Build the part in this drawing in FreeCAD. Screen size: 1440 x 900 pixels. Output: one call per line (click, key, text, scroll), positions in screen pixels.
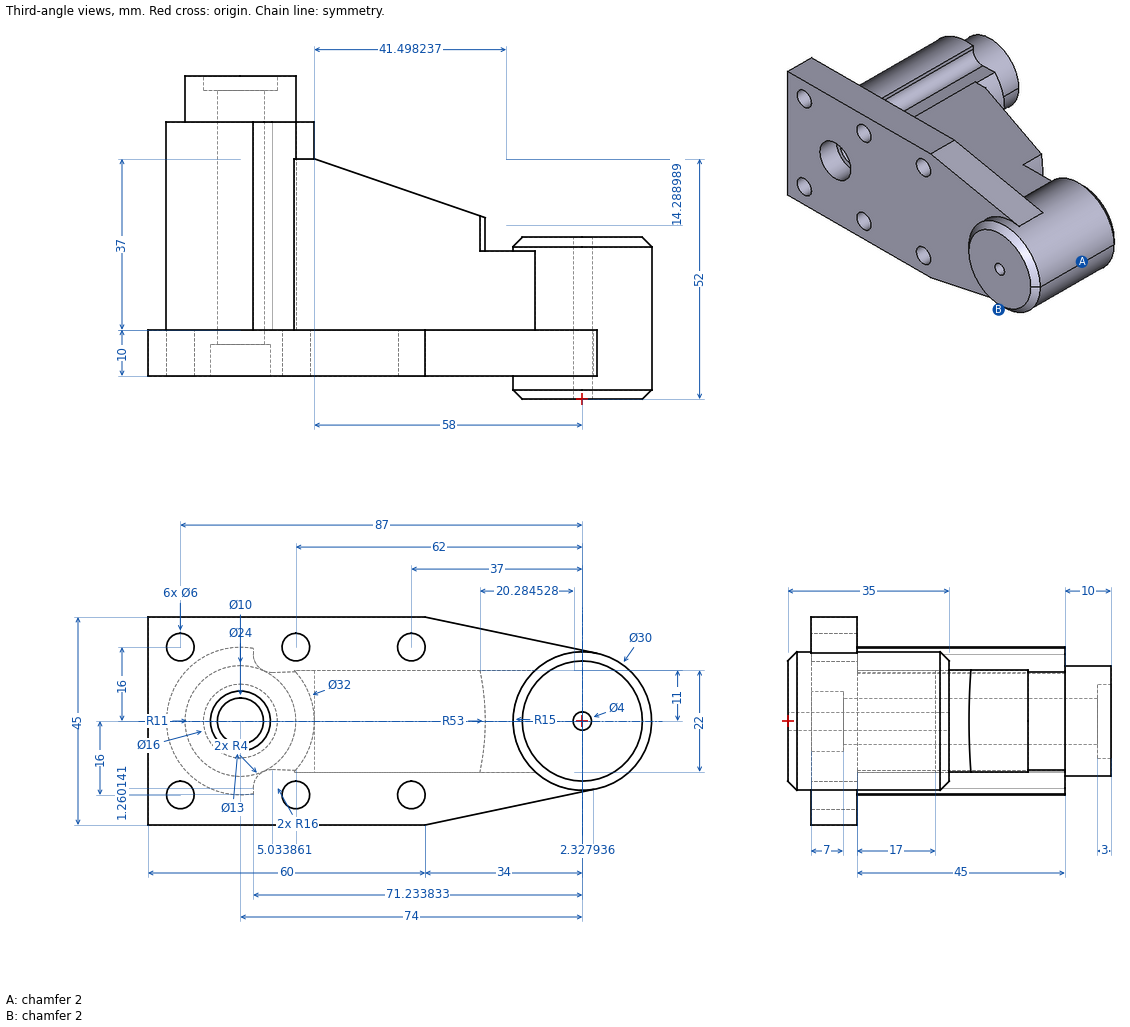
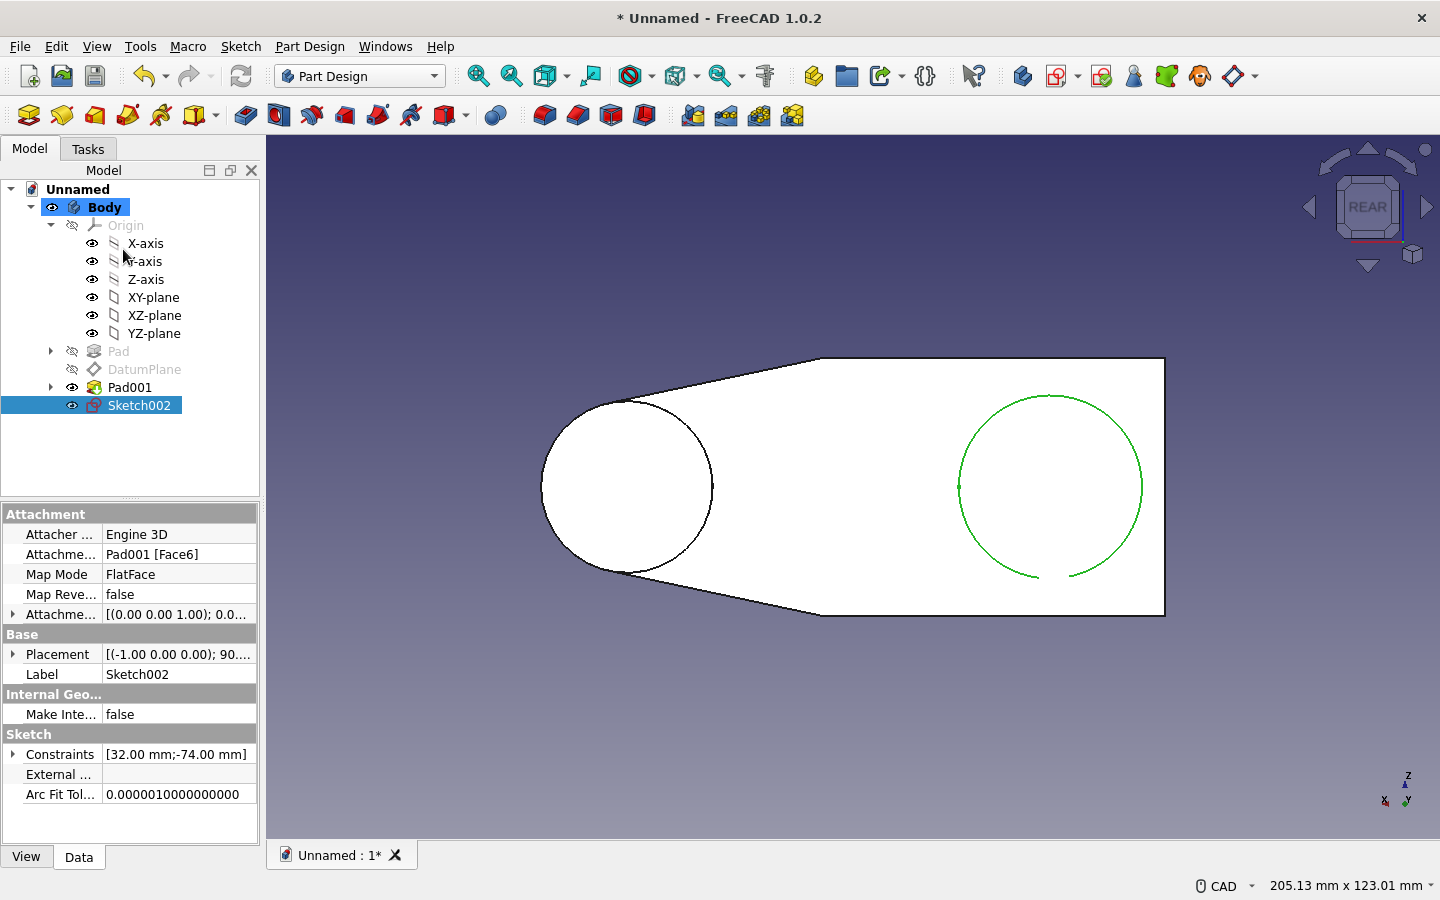
click(29, 116)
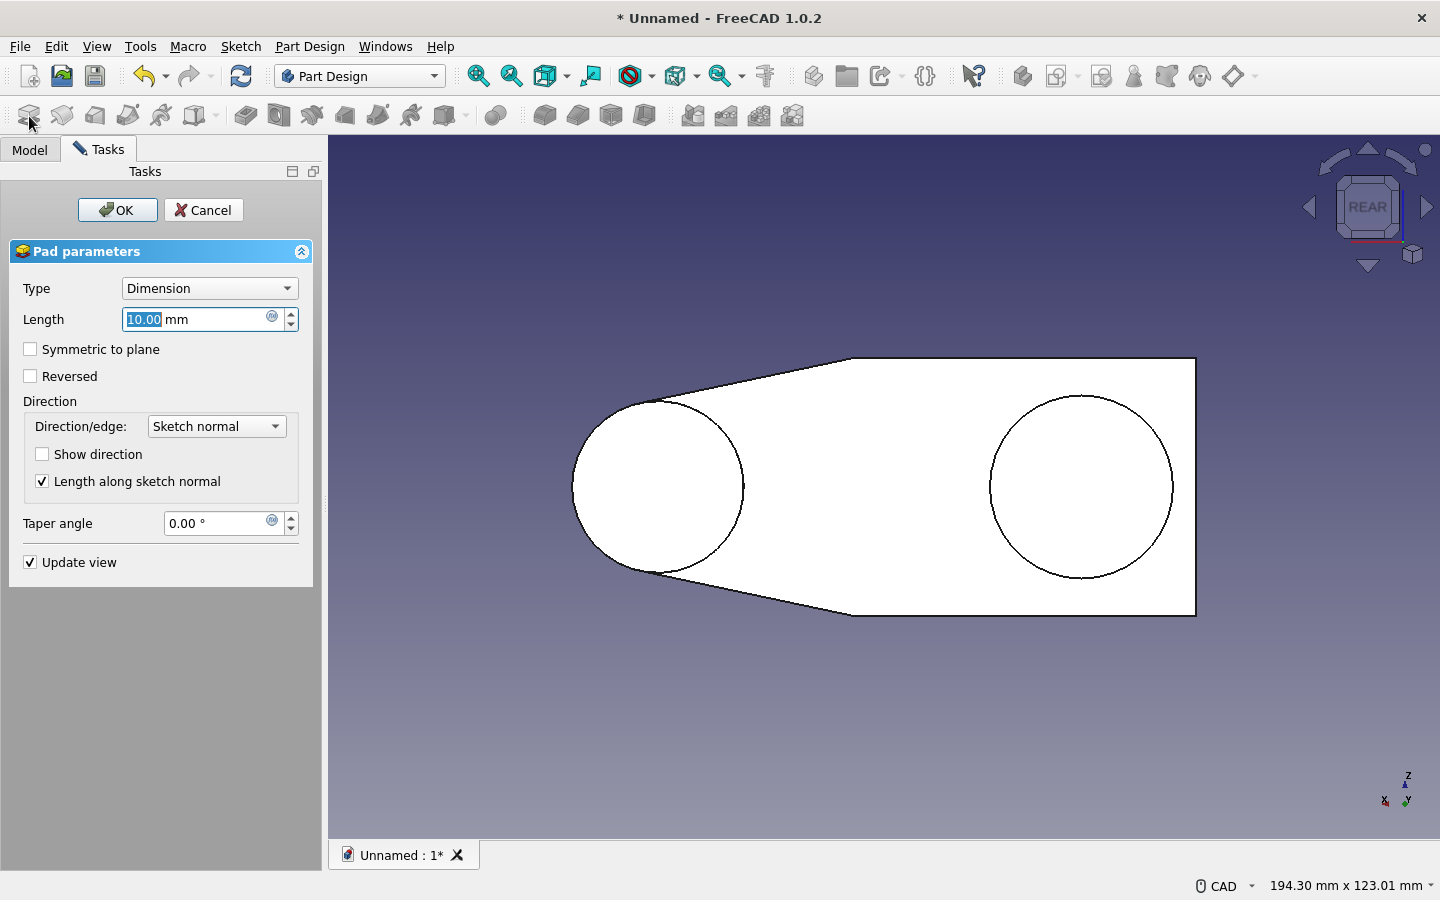
text(45)
key(Tab)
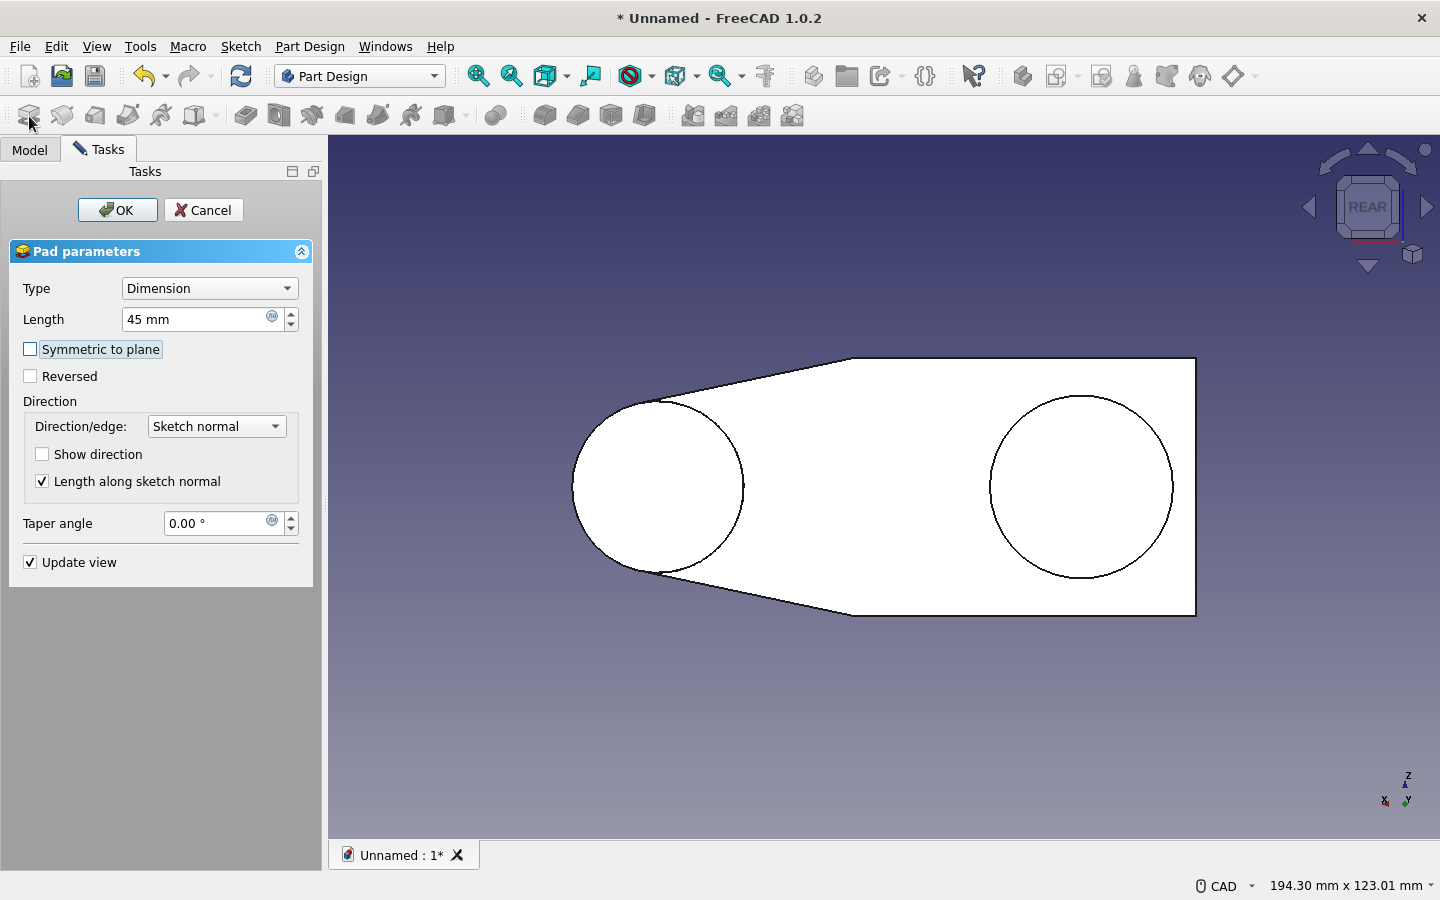
click(118, 210)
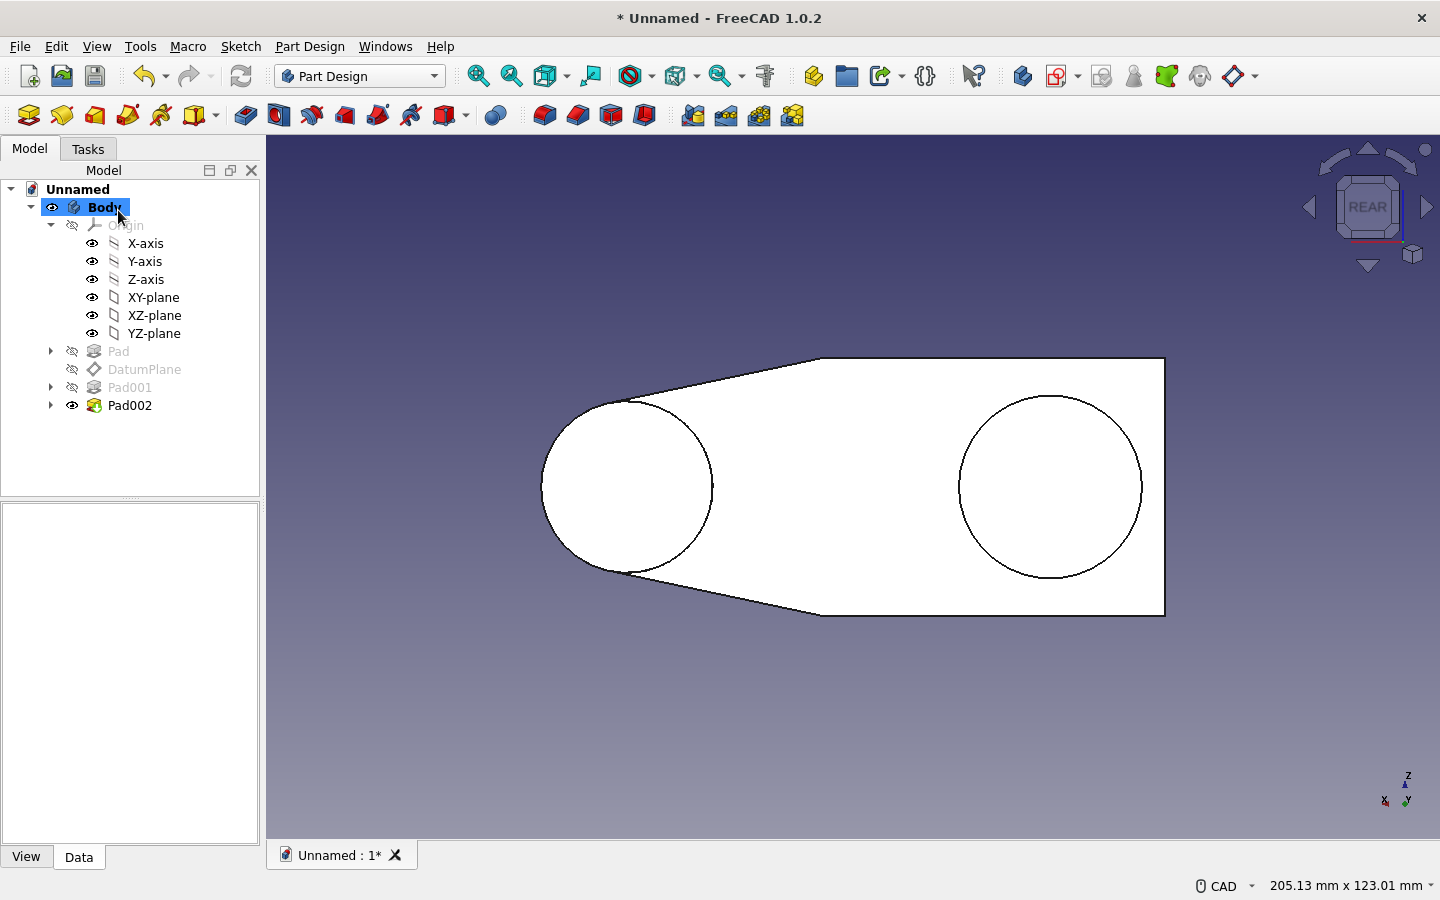
click(808, 486)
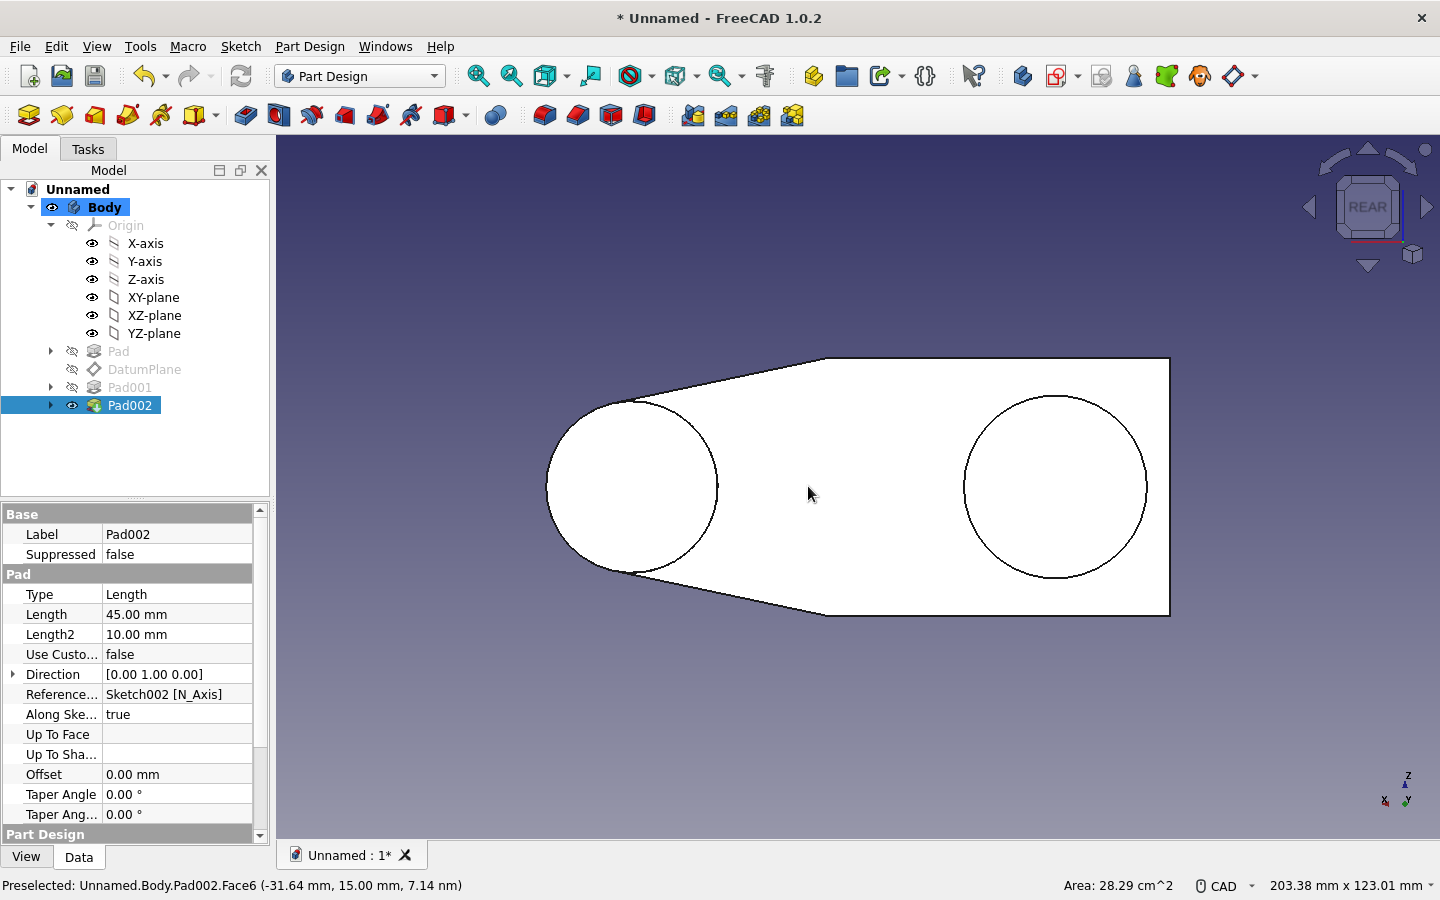
click(1056, 76)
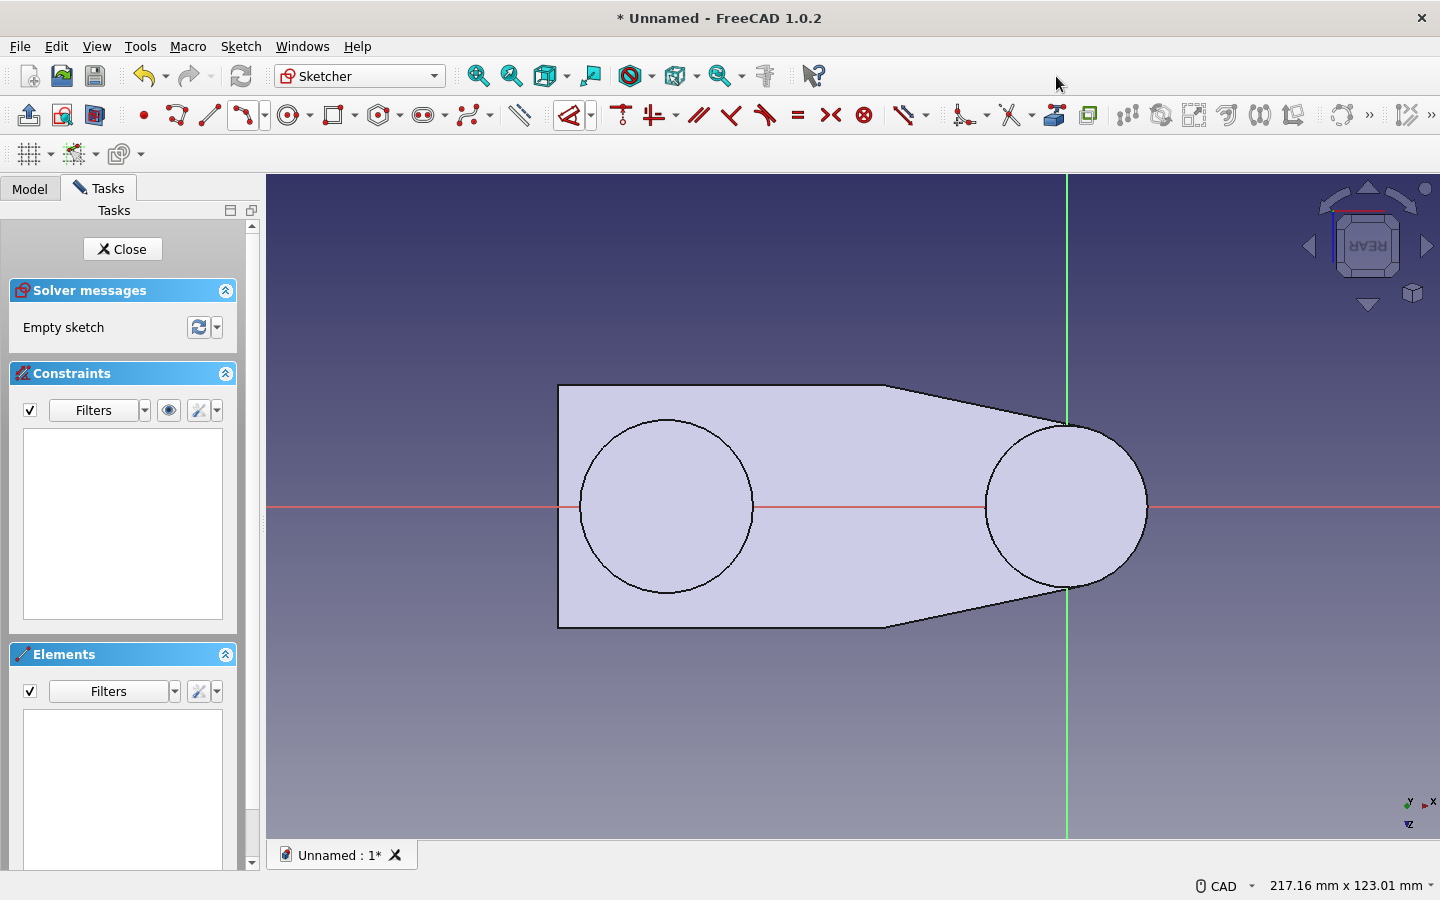
scroll(943, 506, up, 2)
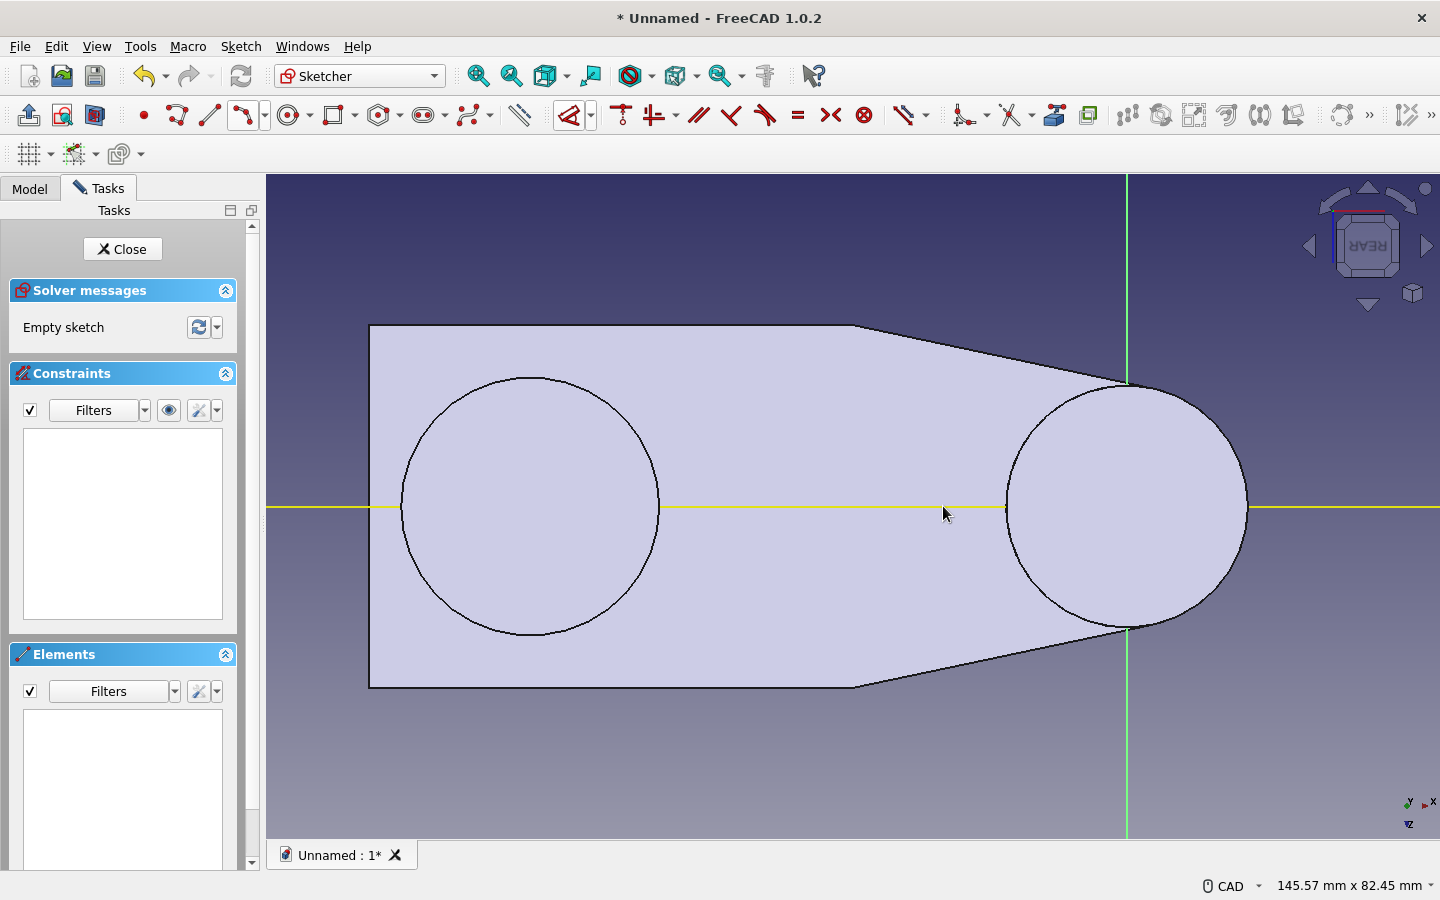
click(210, 116)